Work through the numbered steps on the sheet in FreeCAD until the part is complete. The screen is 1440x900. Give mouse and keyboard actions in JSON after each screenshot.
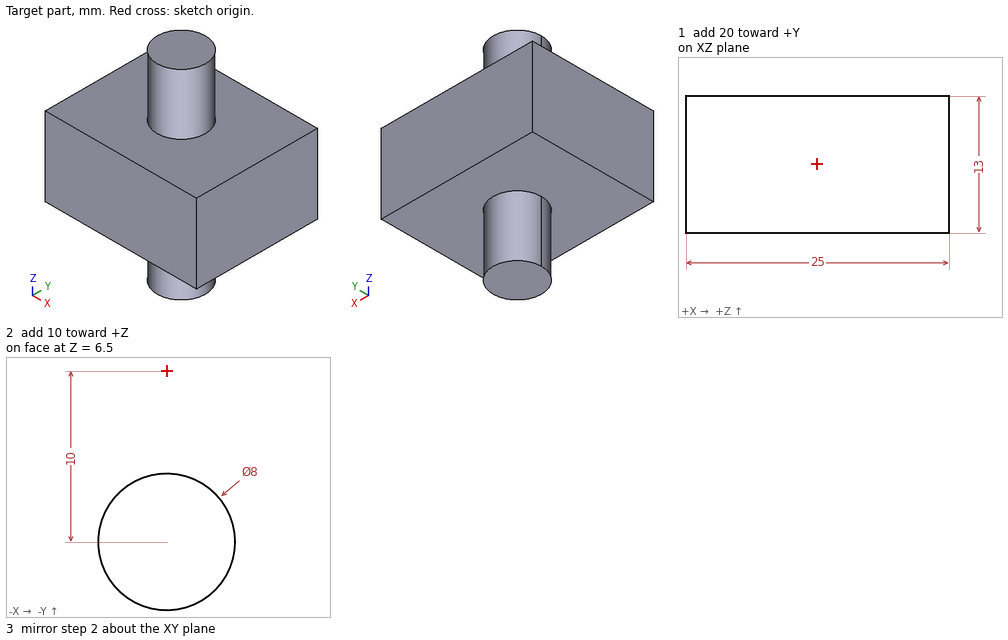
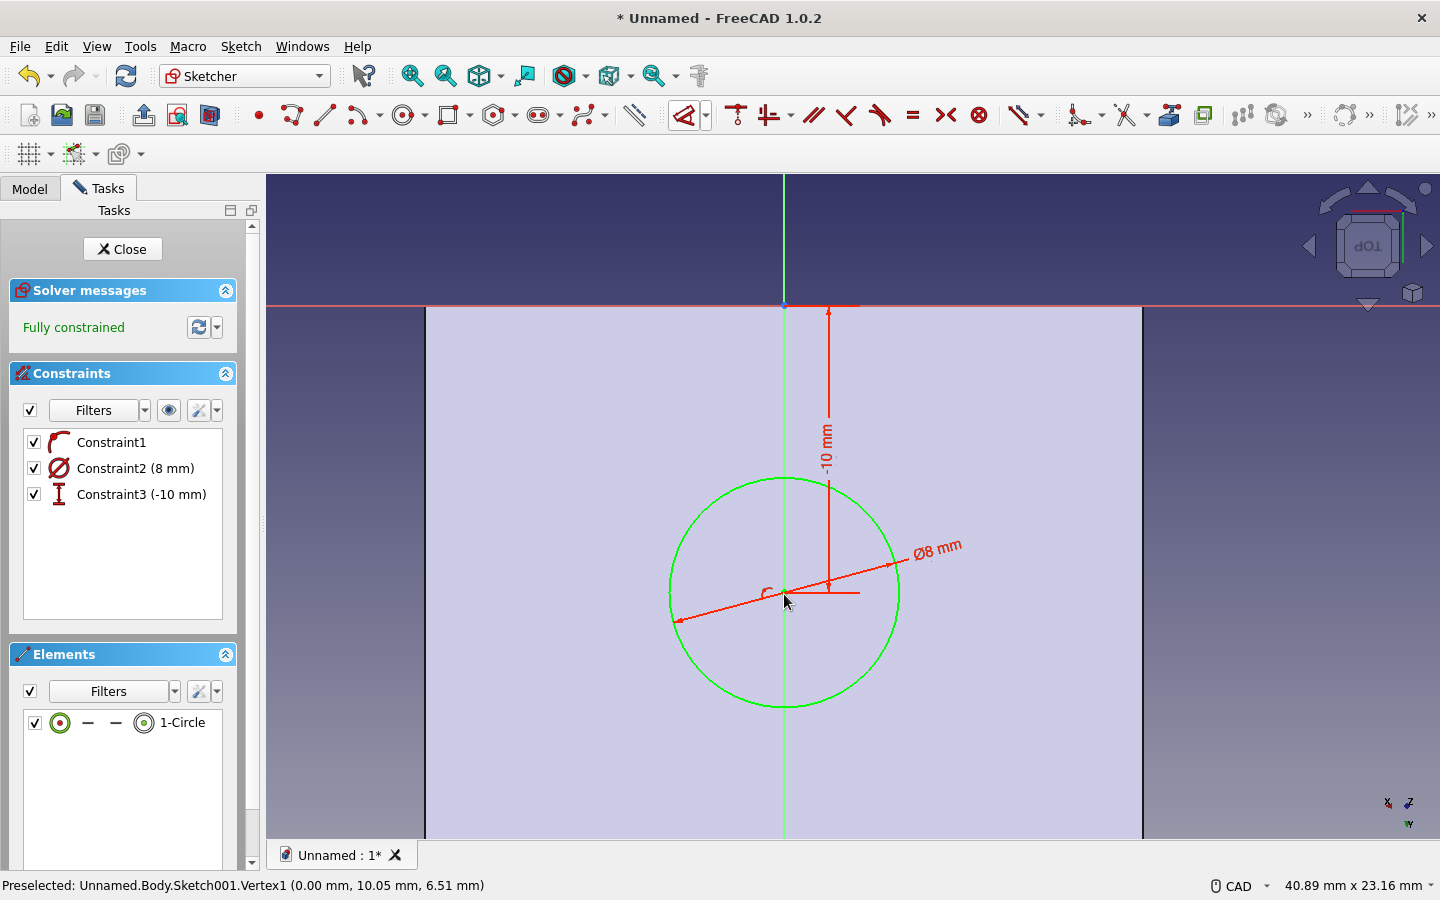
{"action": "left_click", "coordinate": [123, 249]}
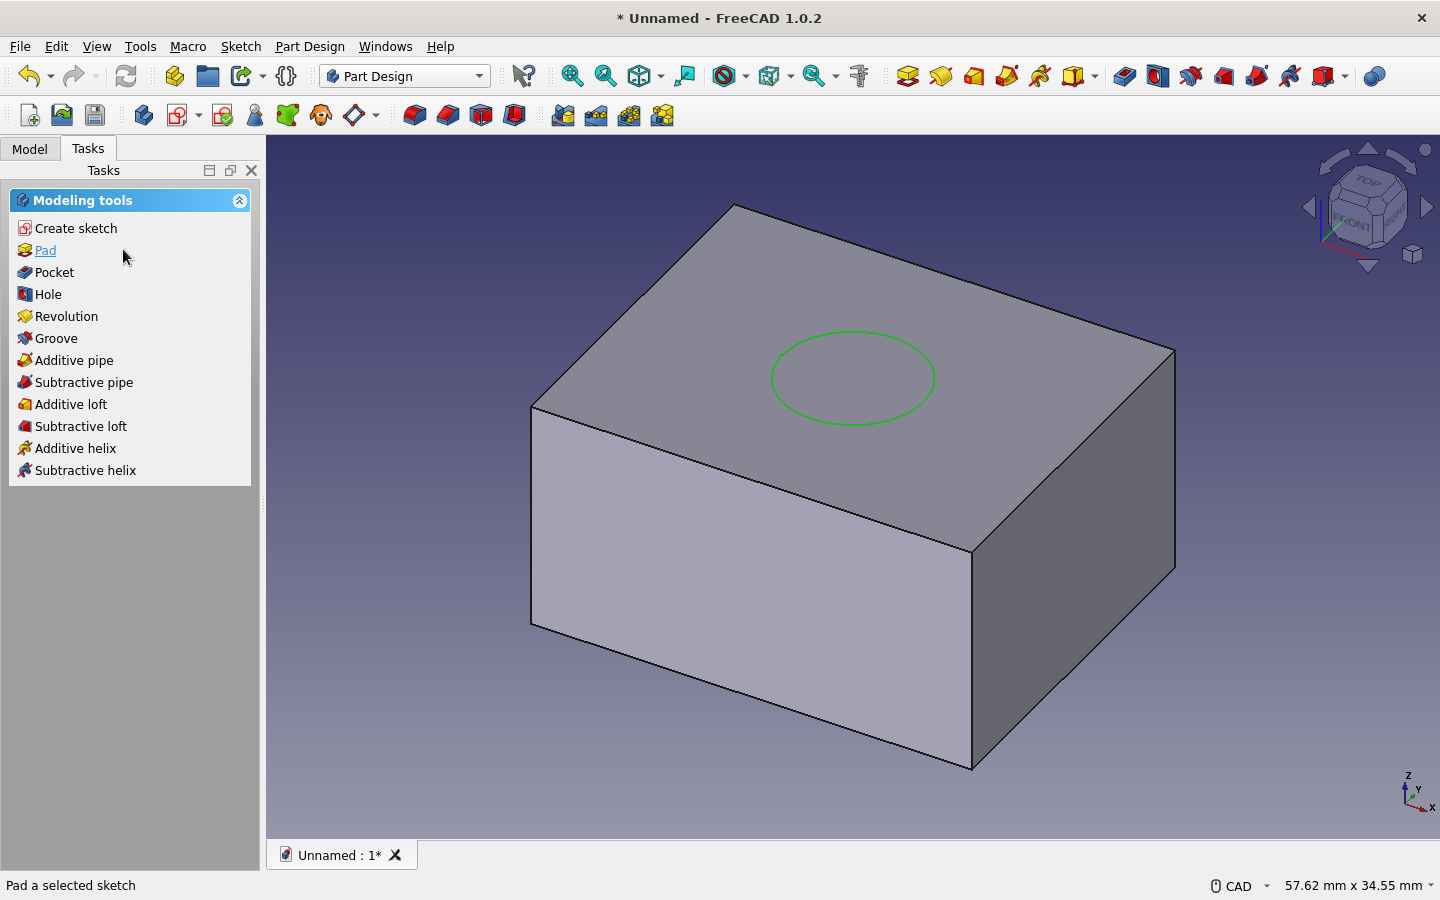
{"action": "left_click", "coordinate": [908, 76]}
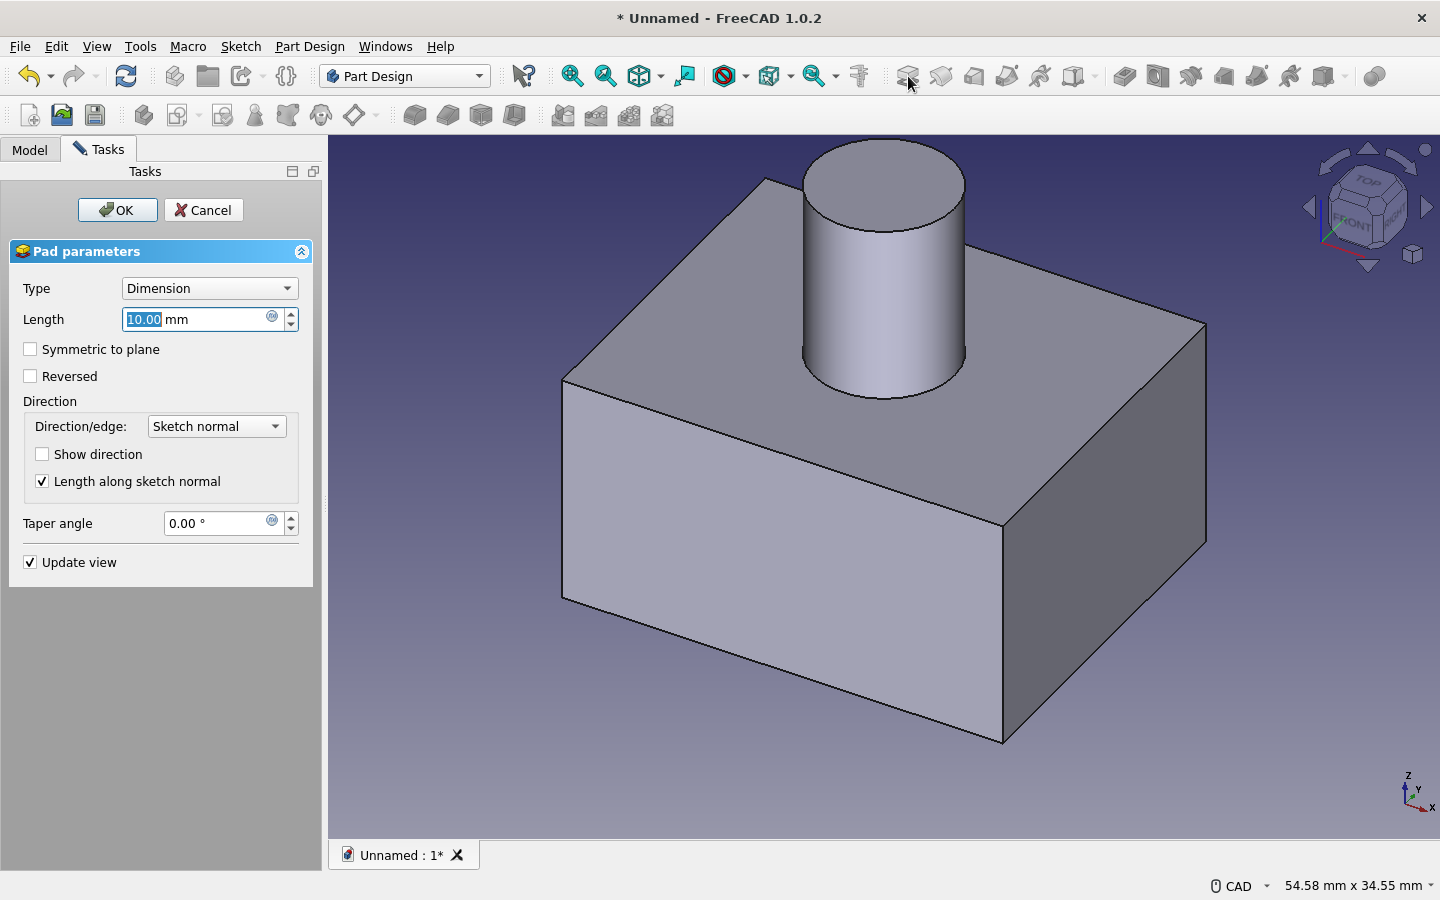
{"action": "type", "text": "10"}
{"action": "key", "text": "Tab"}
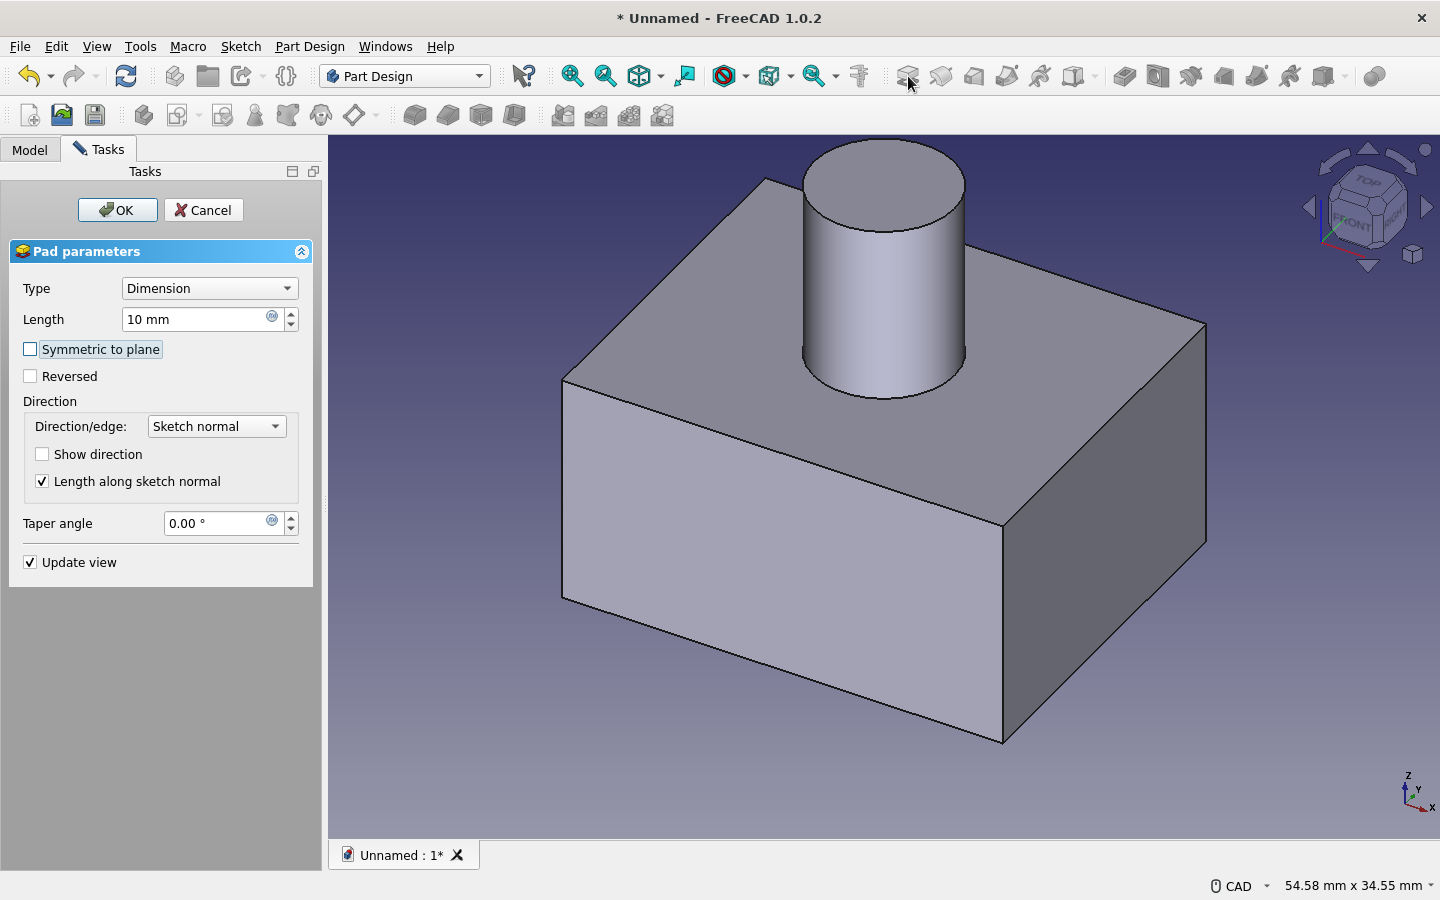
{"action": "left_click", "coordinate": [118, 210]}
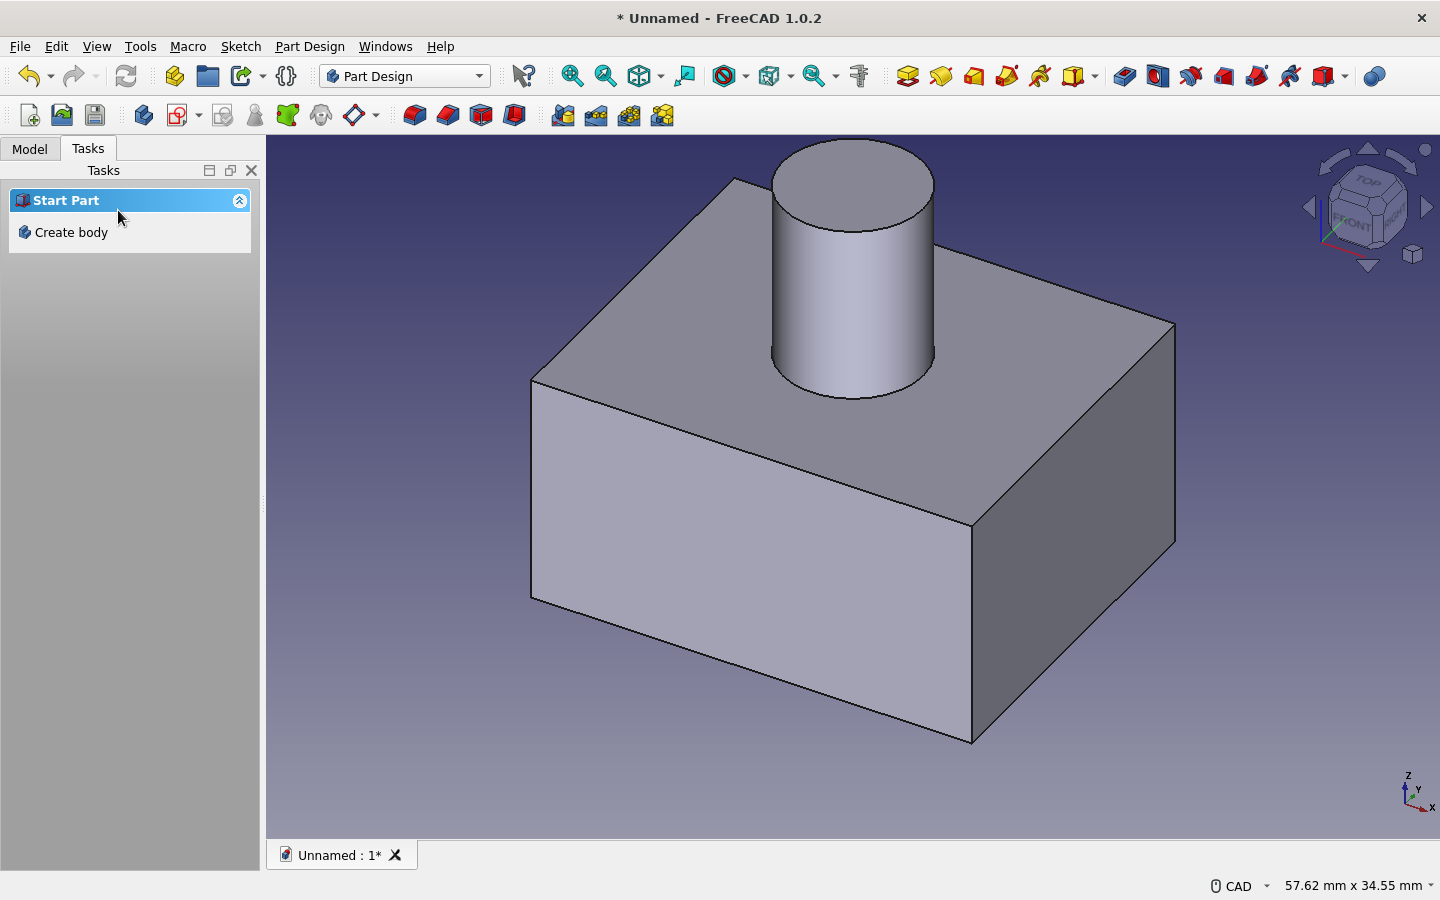
{"action": "left_click", "coordinate": [573, 76]}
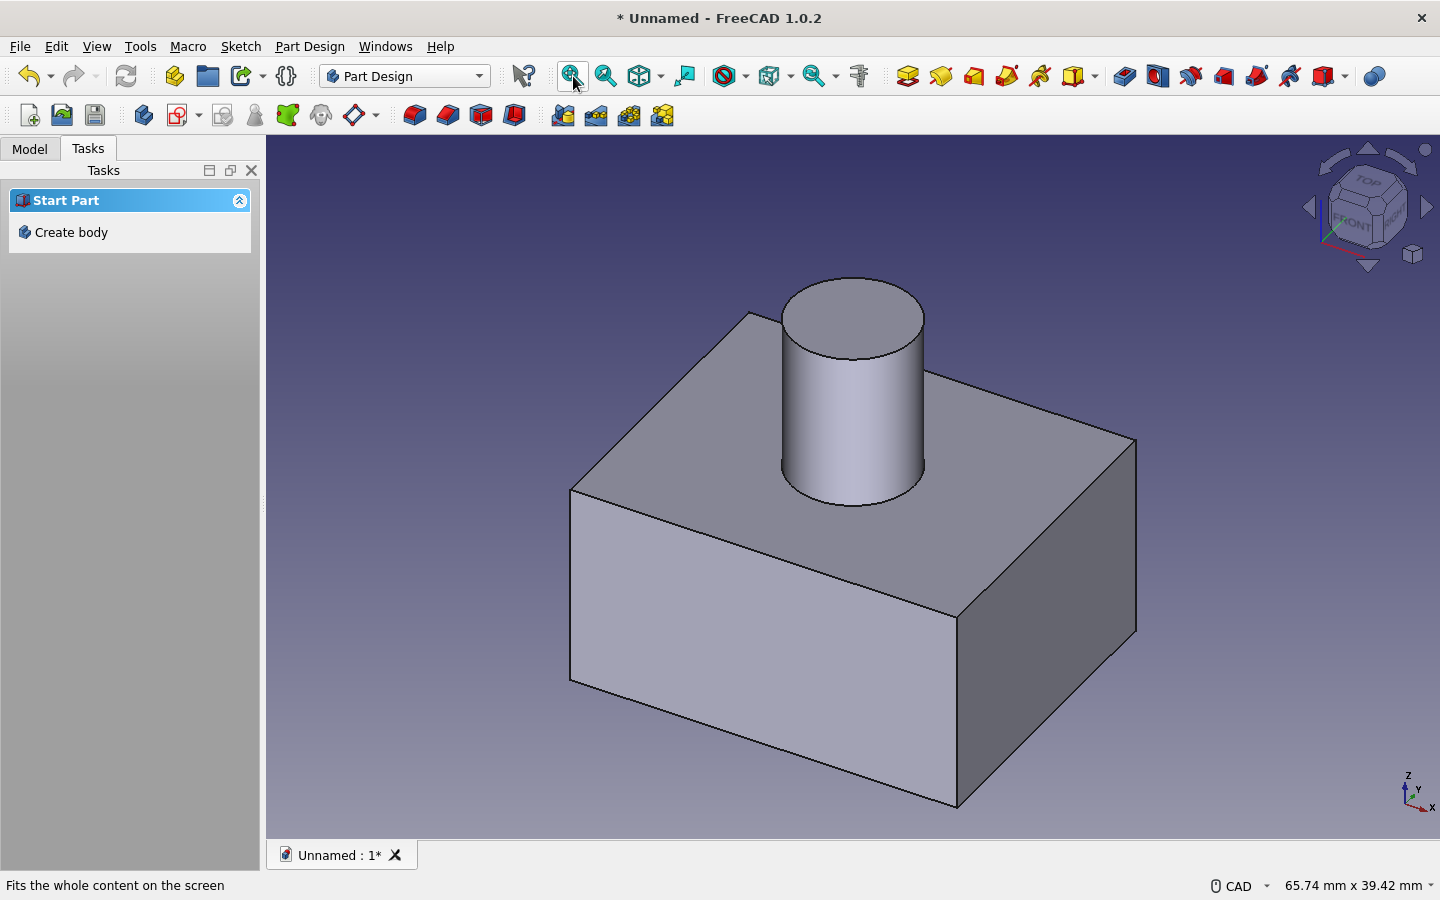
{"action": "left_click", "coordinate": [30, 148]}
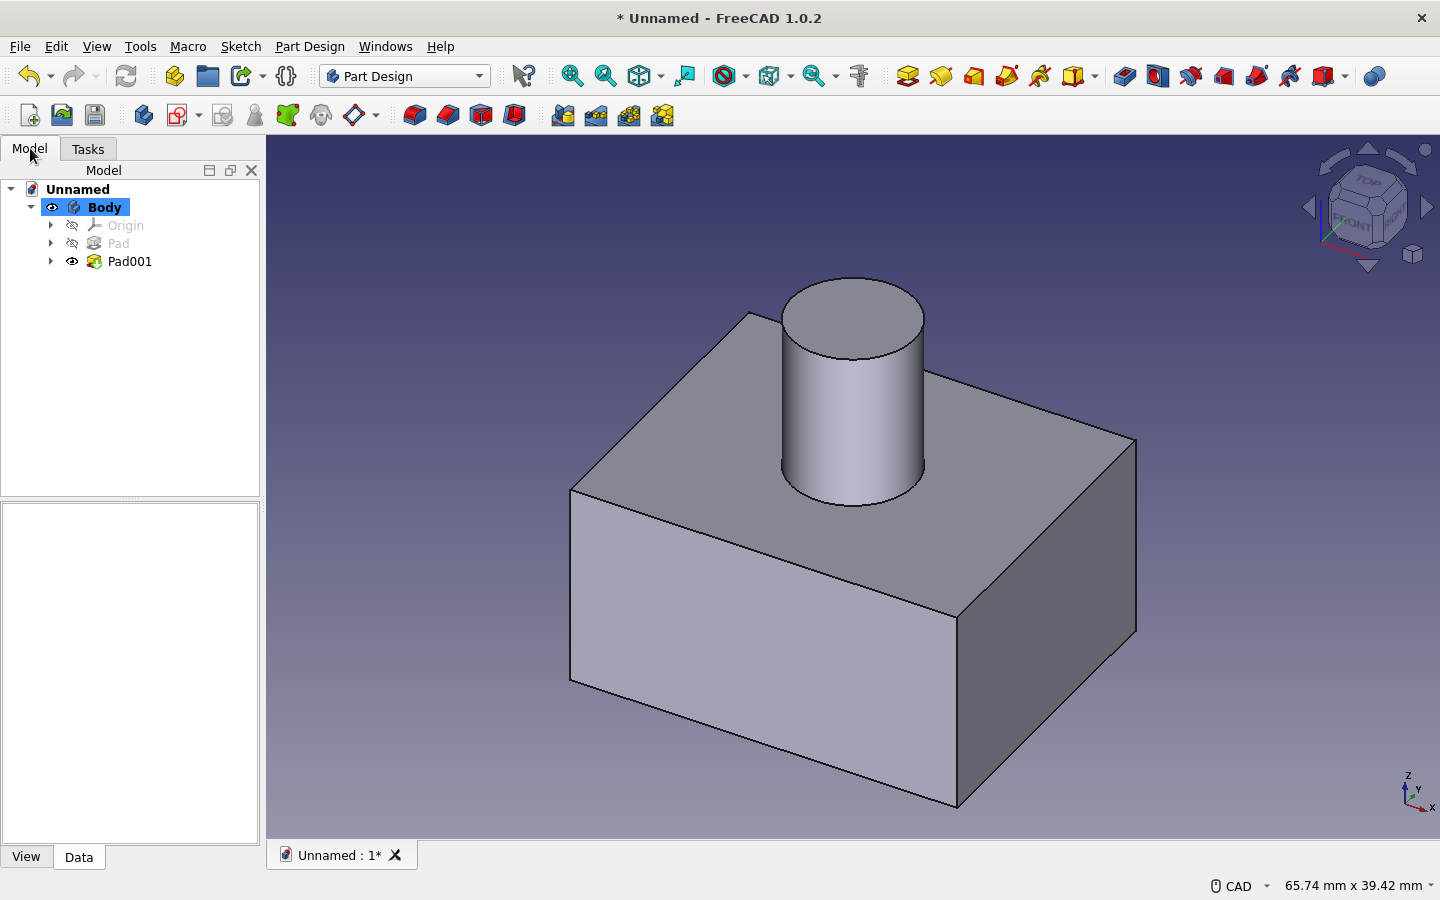
{"action": "left_click", "coordinate": [117, 261]}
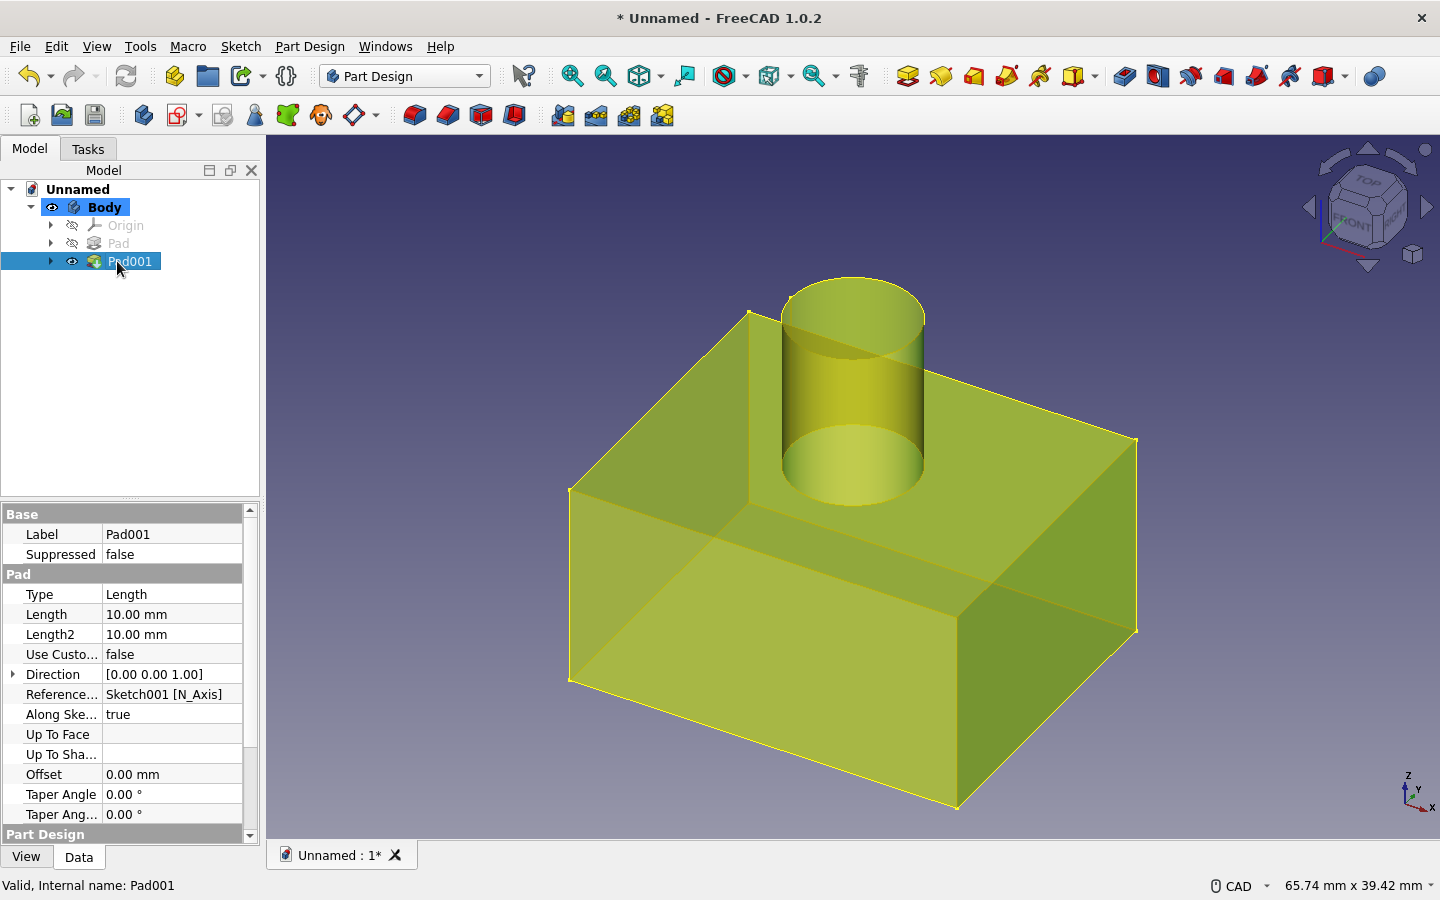
{"action": "left_click", "coordinate": [563, 116]}